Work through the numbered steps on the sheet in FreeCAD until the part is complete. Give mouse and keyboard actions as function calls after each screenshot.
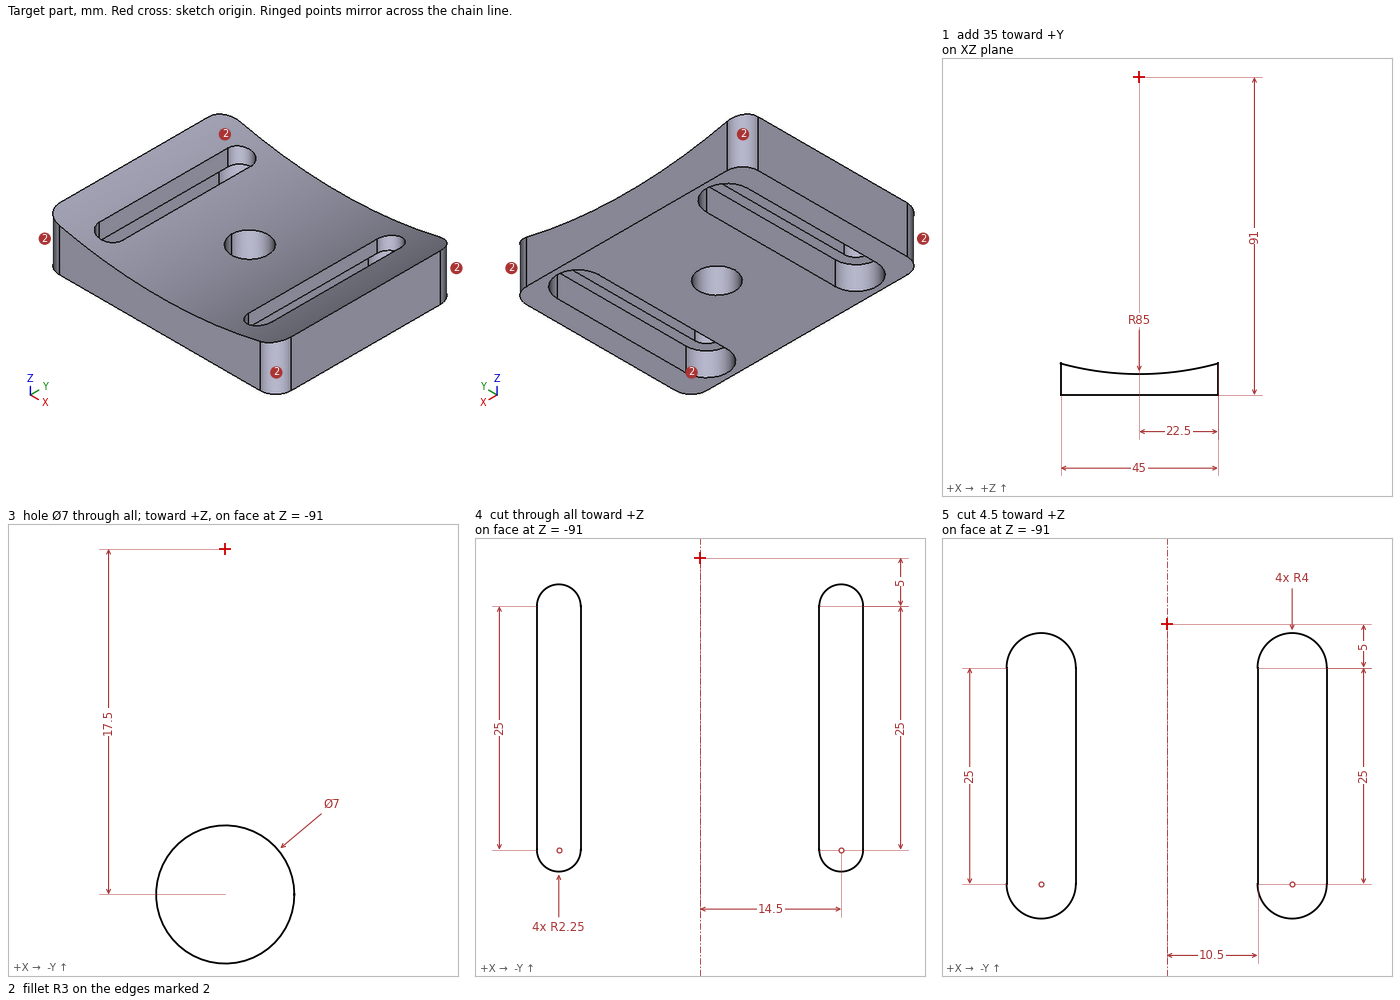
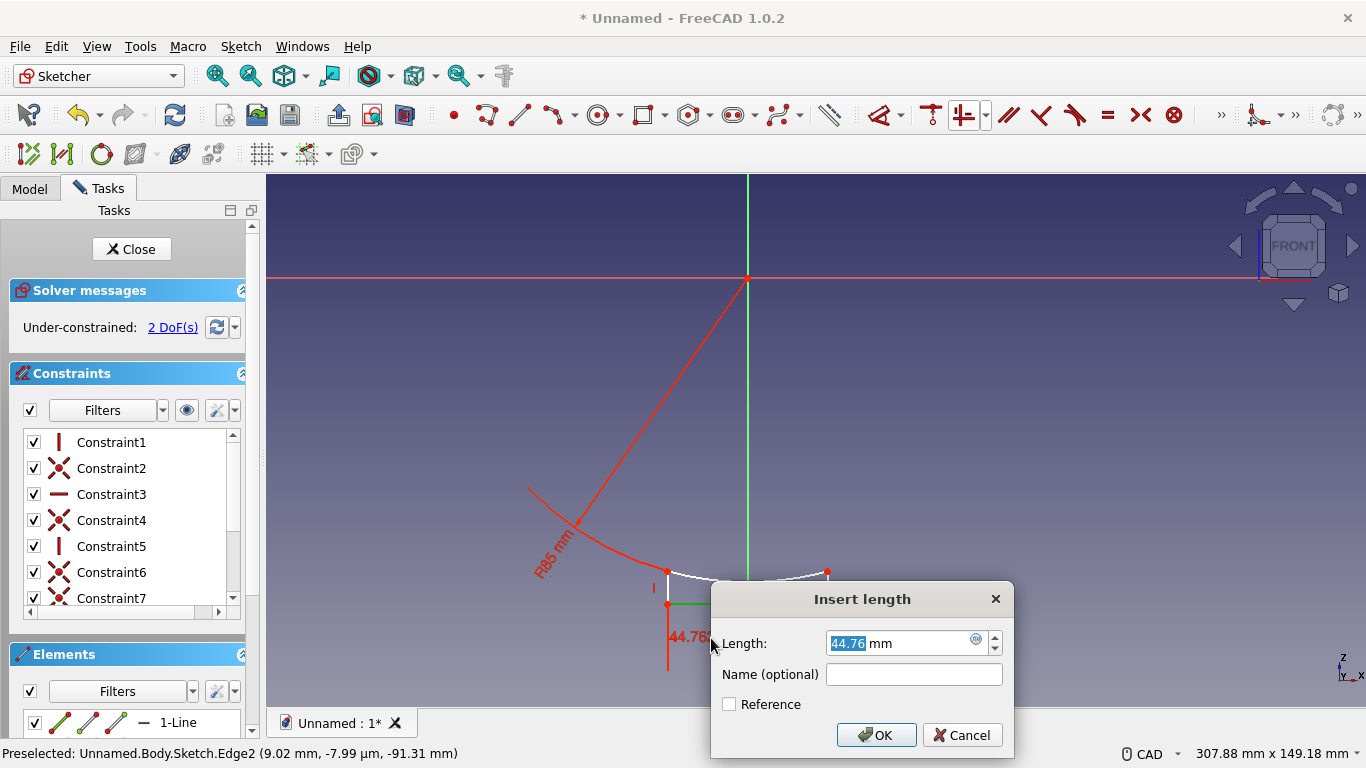
text(45)
key(Return)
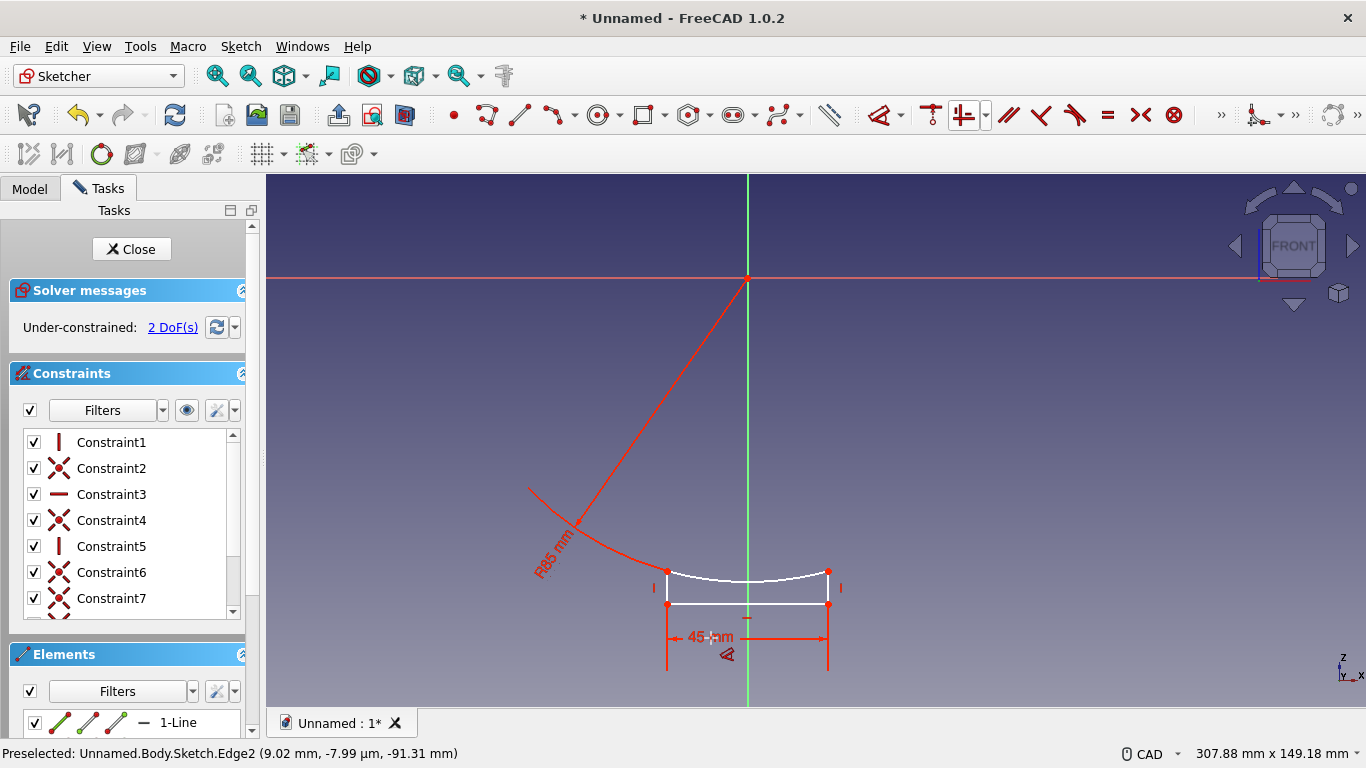
click(828, 604)
click(862, 441)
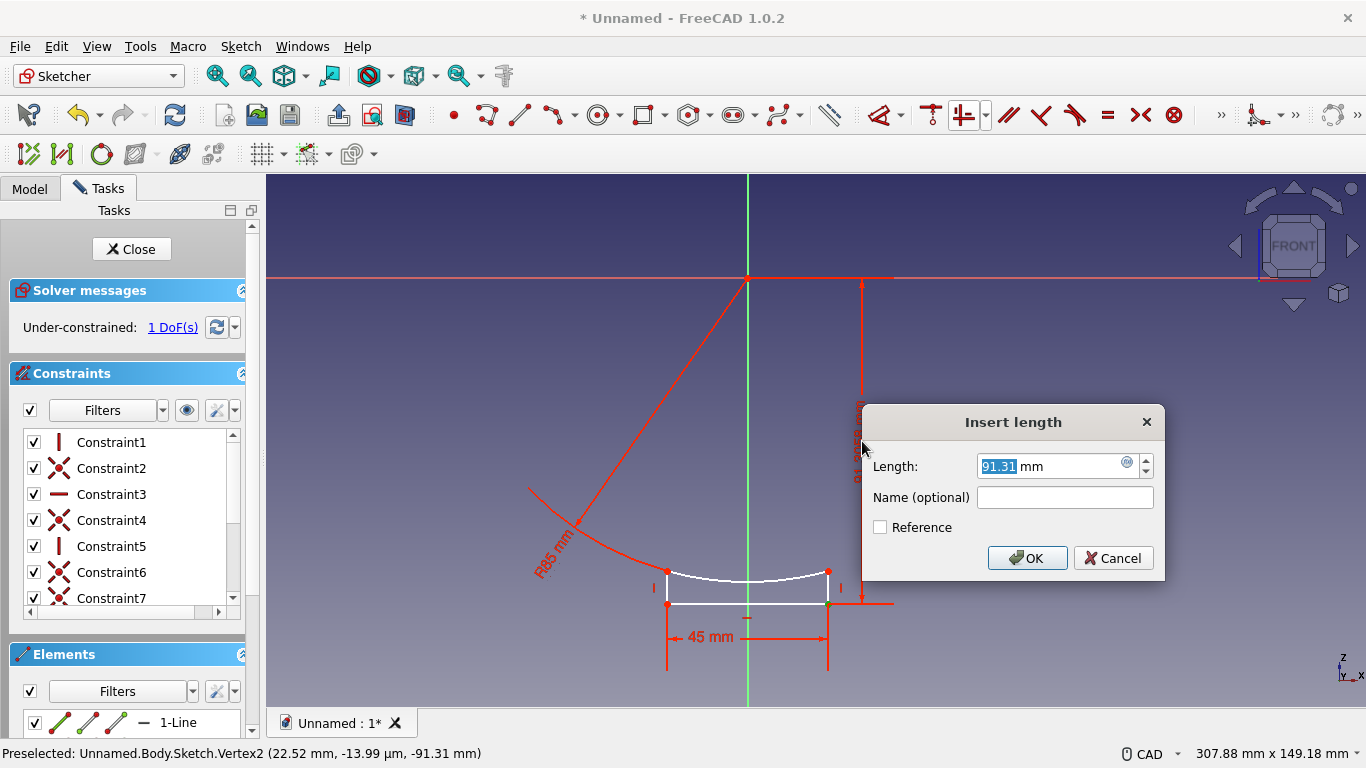
text(91)
key(Return)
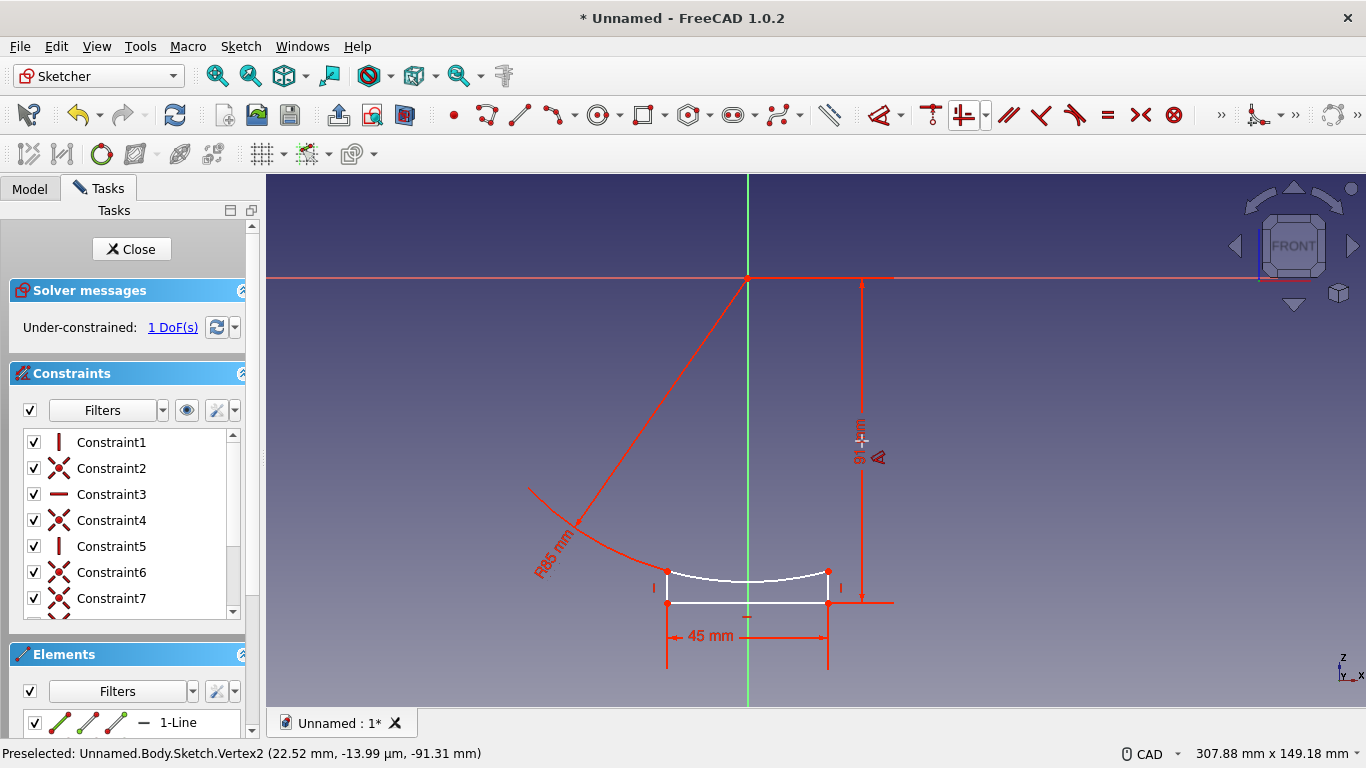
click(828, 571)
click(788, 244)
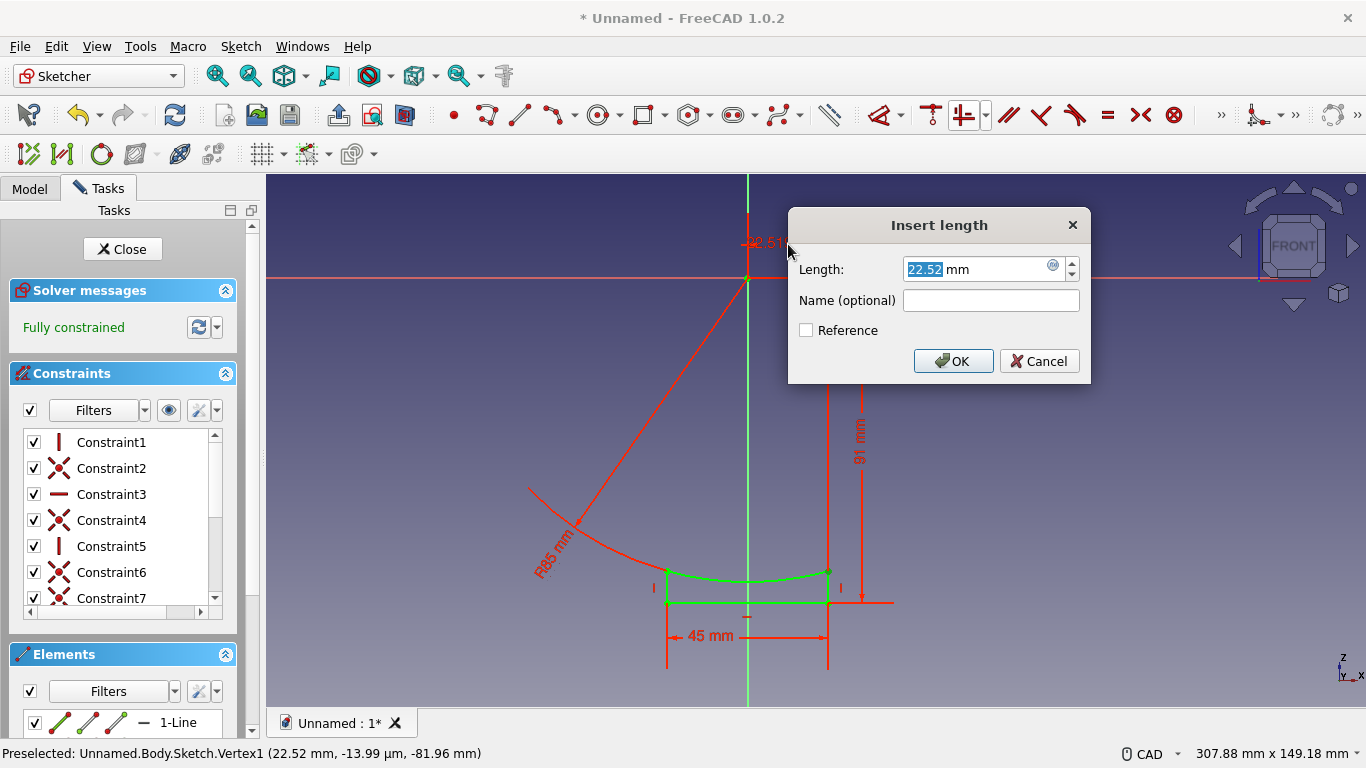
text(22.5)
key(Return)
key(Escape)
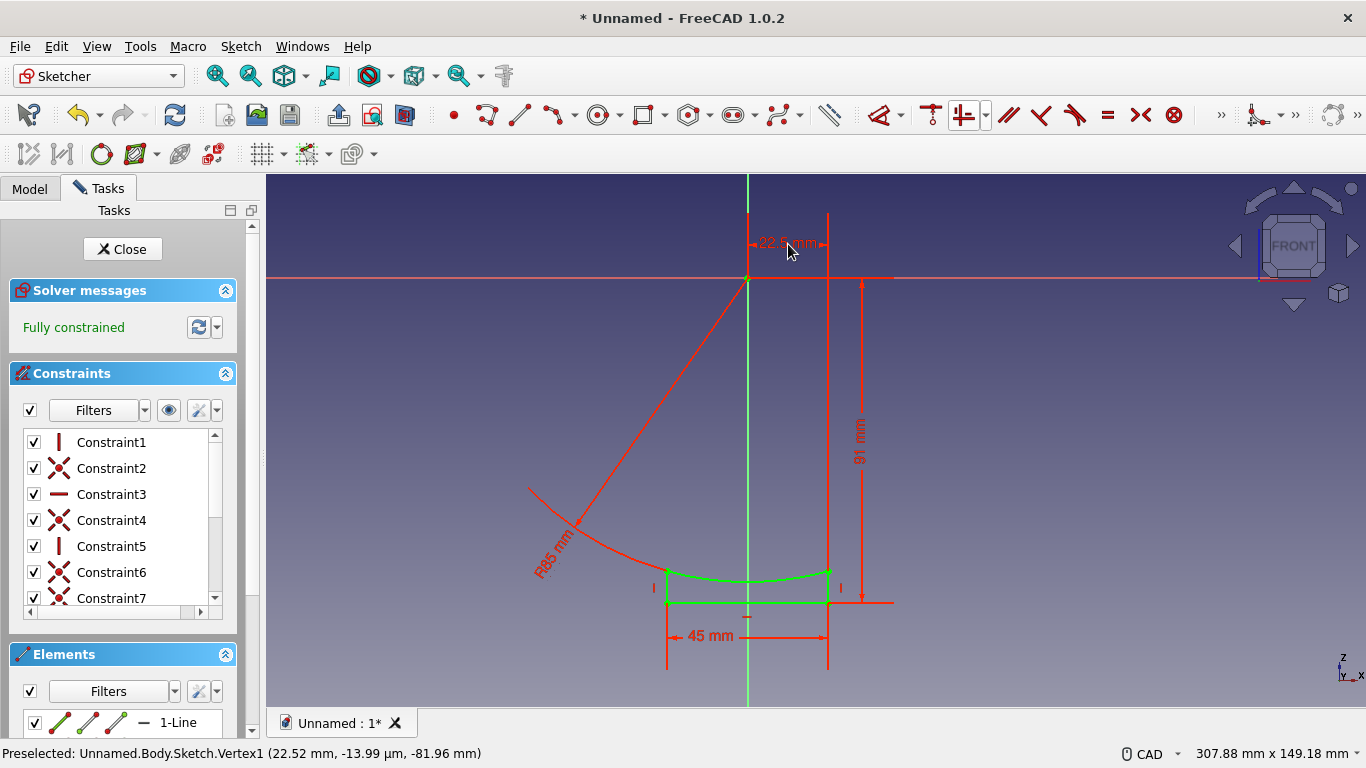
click(123, 249)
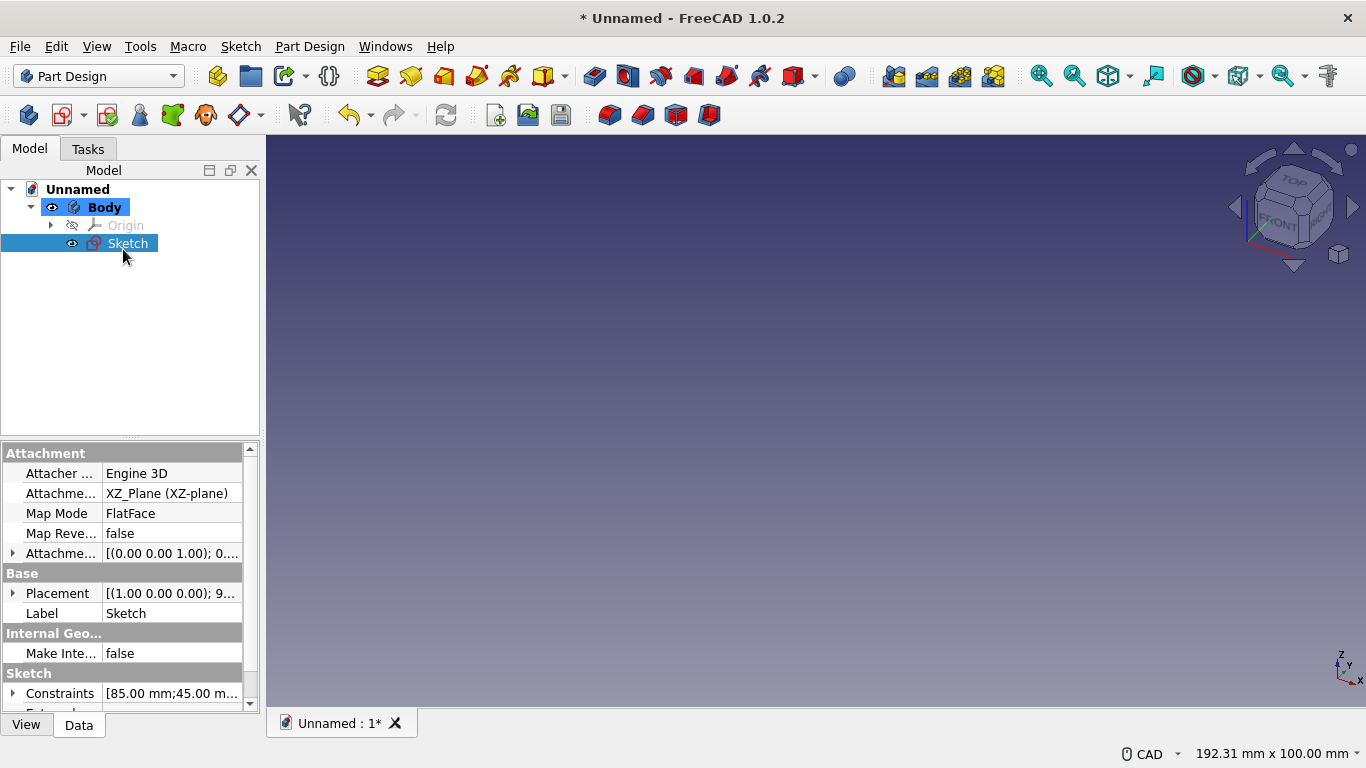
click(378, 76)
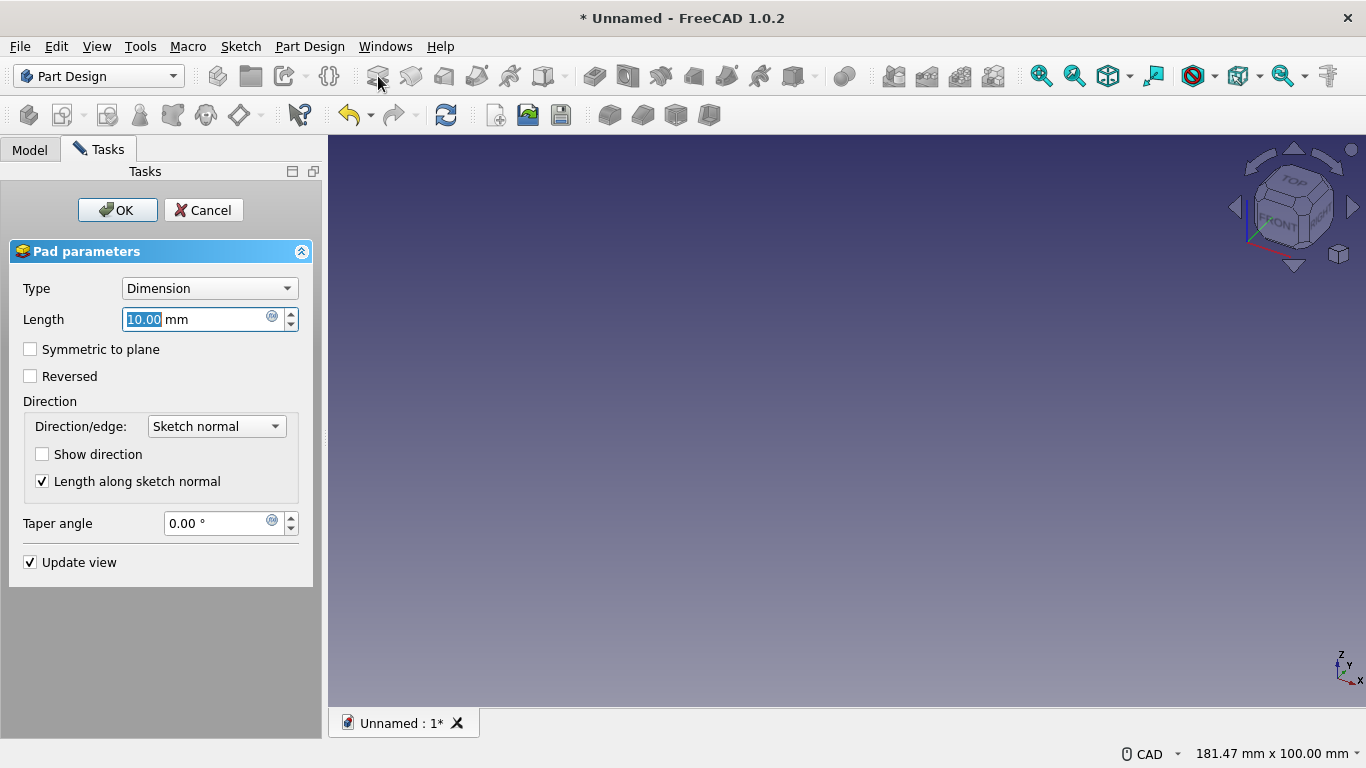
text(35)
key(Tab)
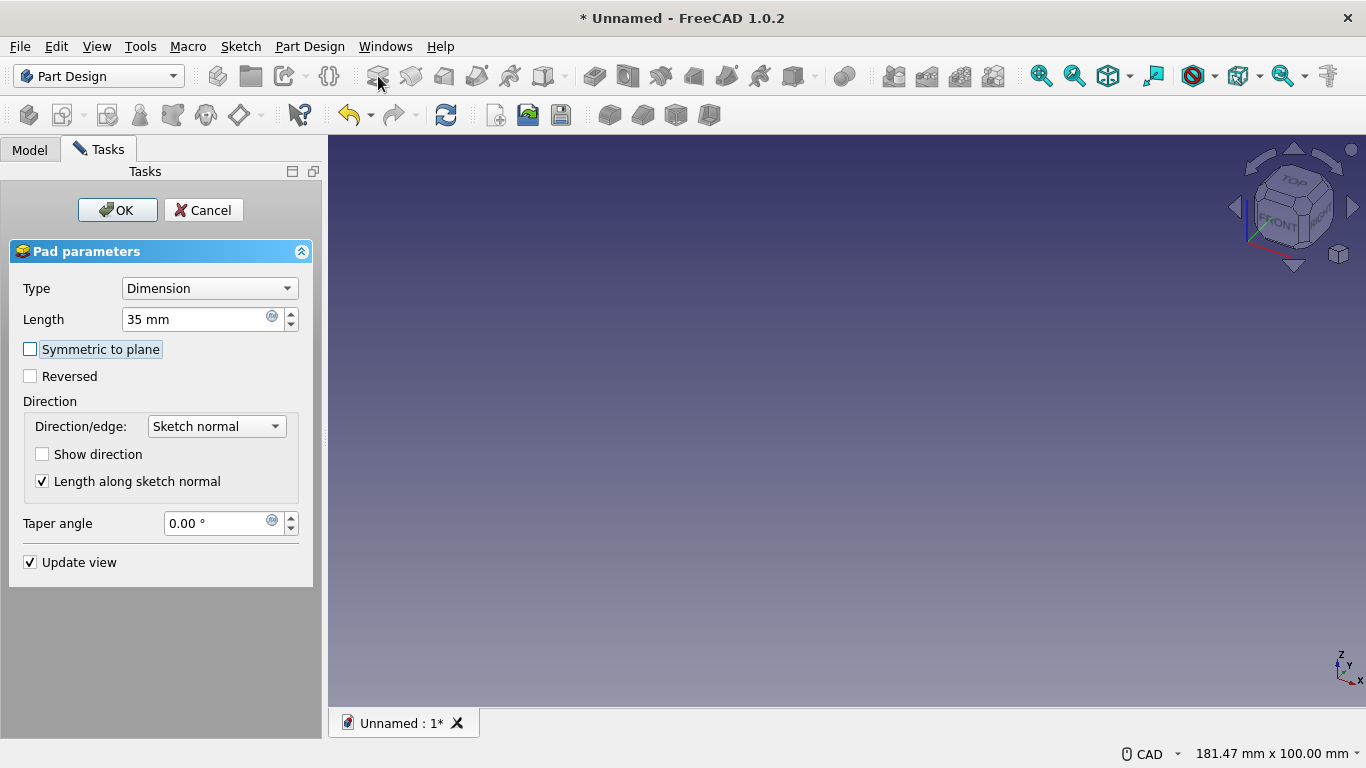
click(31, 376)